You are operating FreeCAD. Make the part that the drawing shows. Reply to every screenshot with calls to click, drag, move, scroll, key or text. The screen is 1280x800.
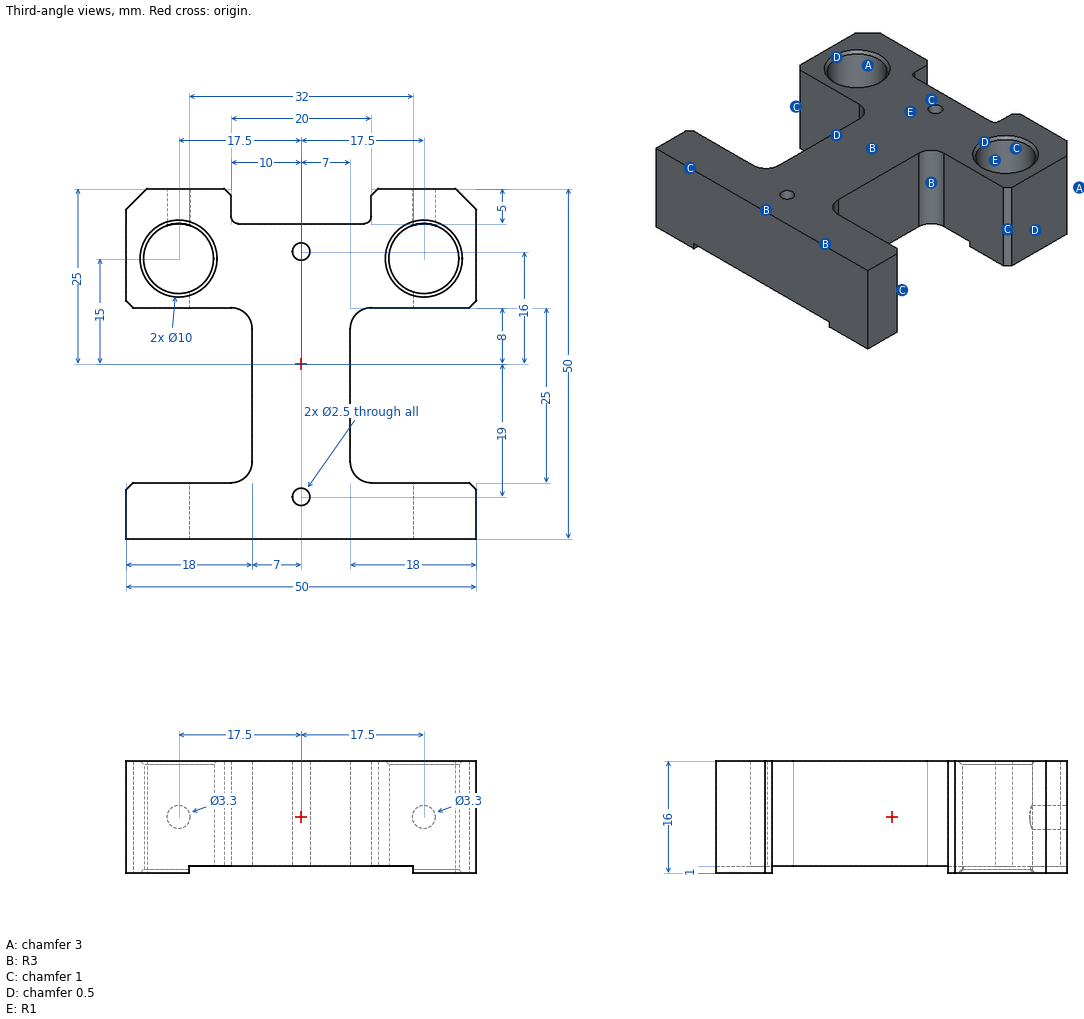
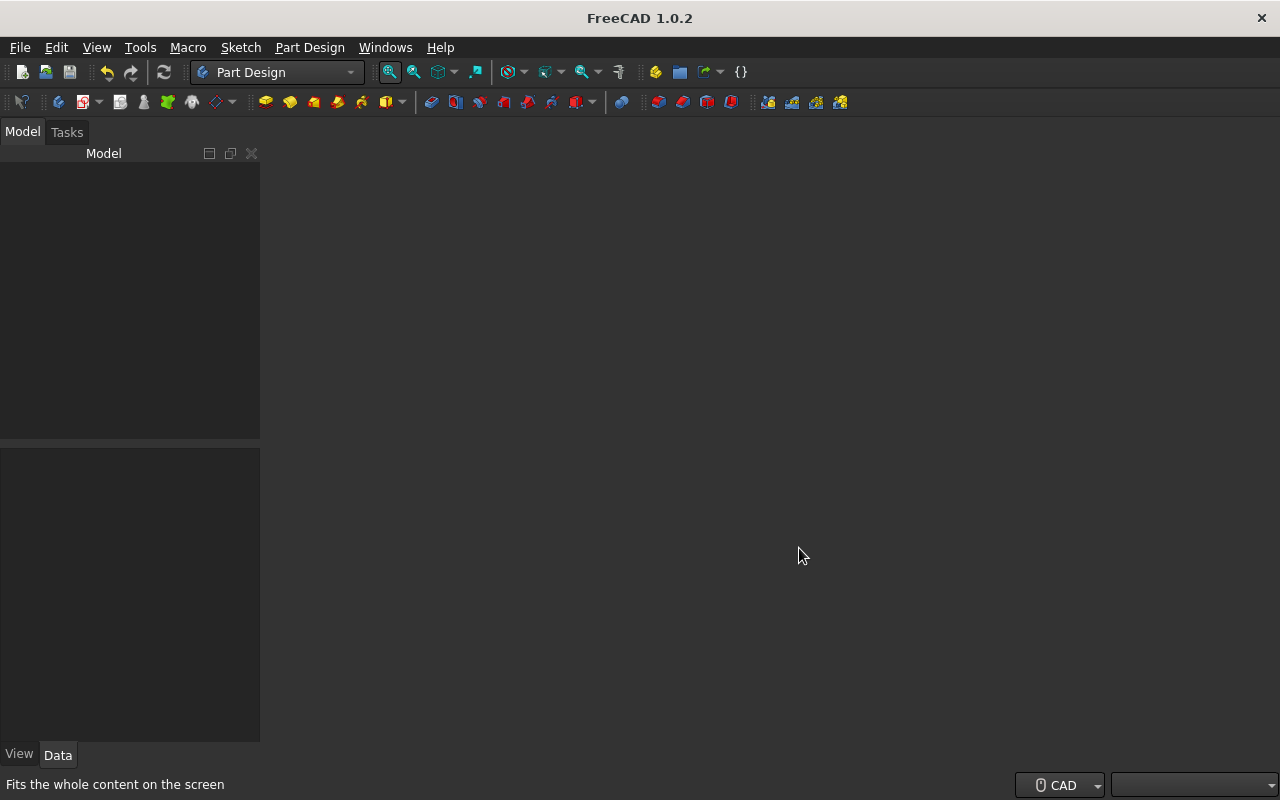
click(22, 72)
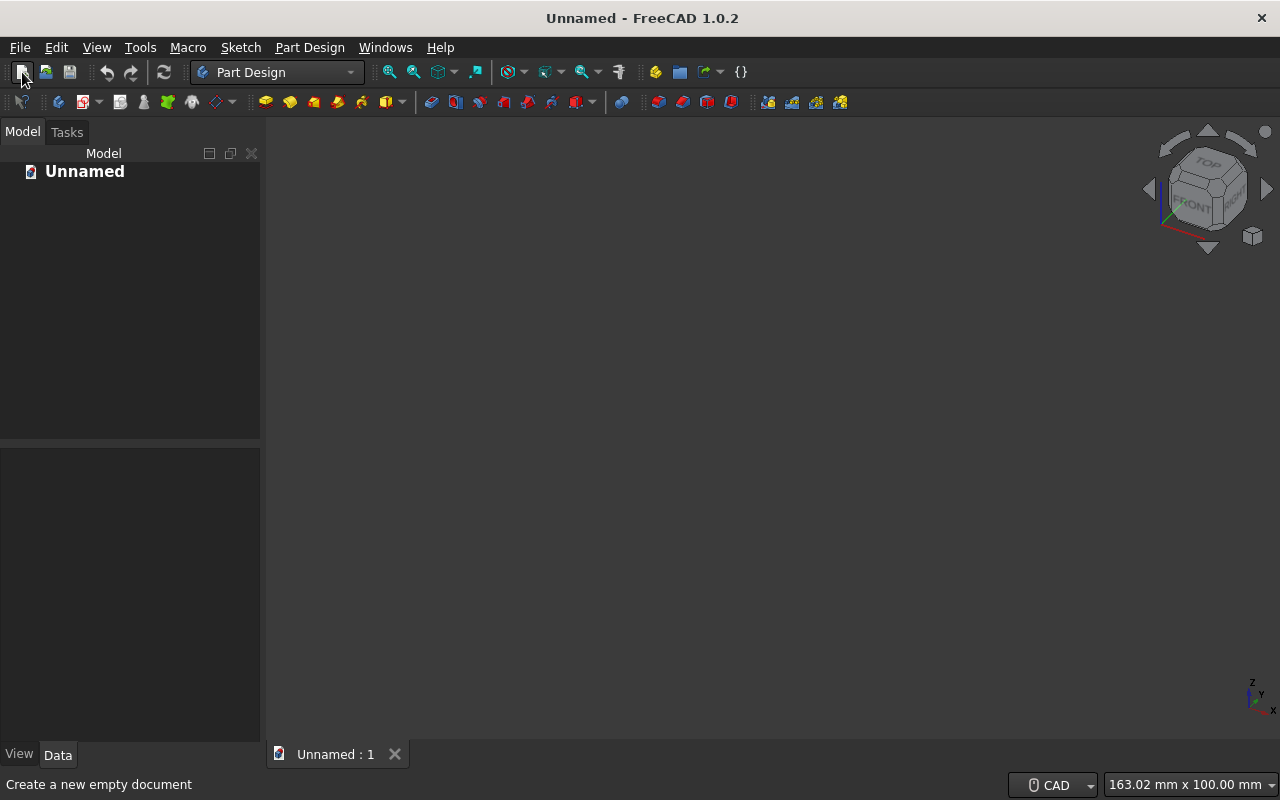
click(84, 102)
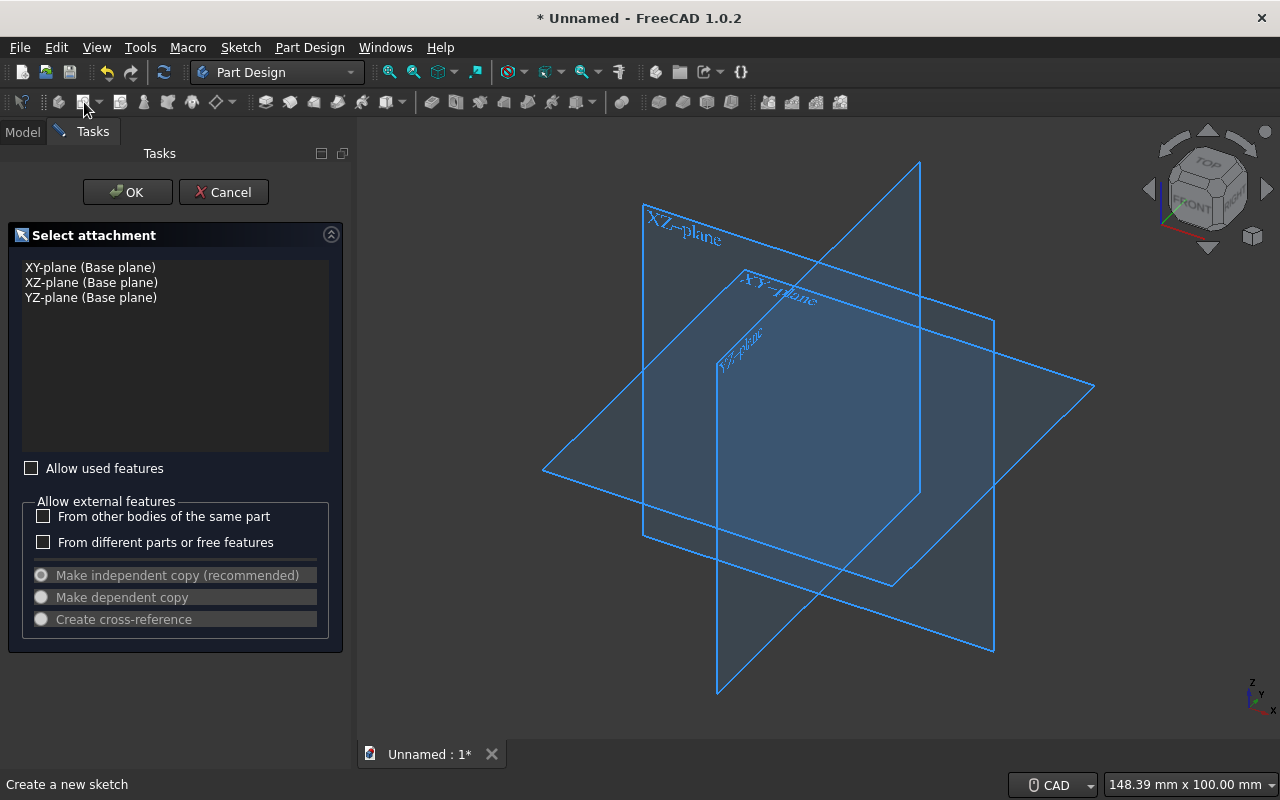
click(82, 268)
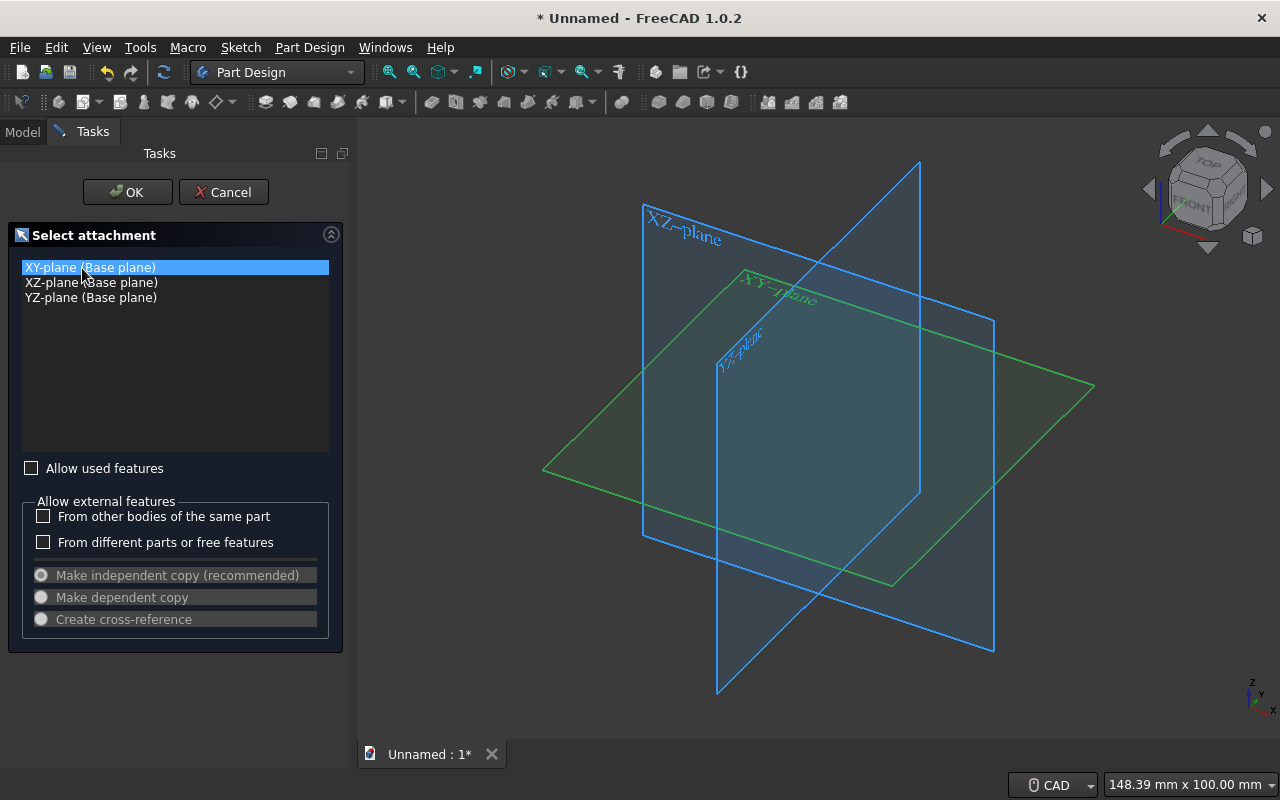
click(128, 192)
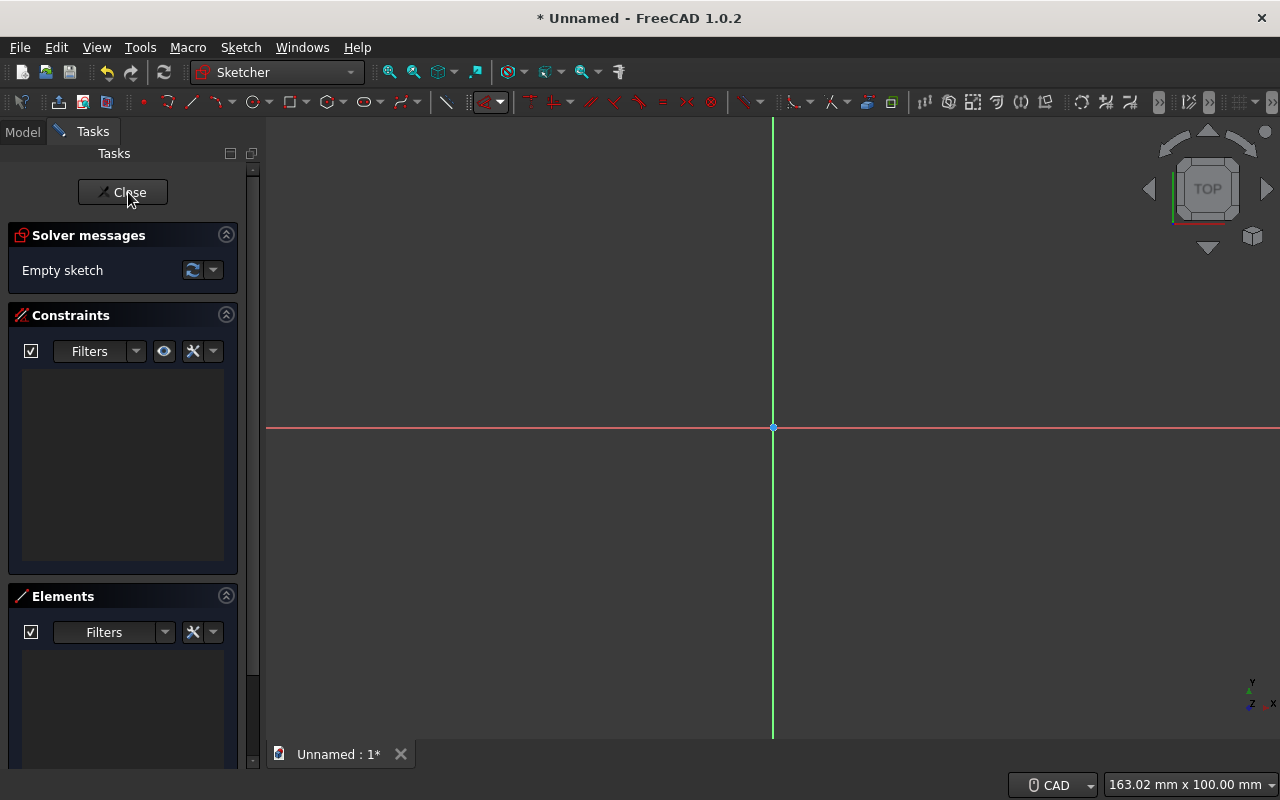
key(g)
key(v)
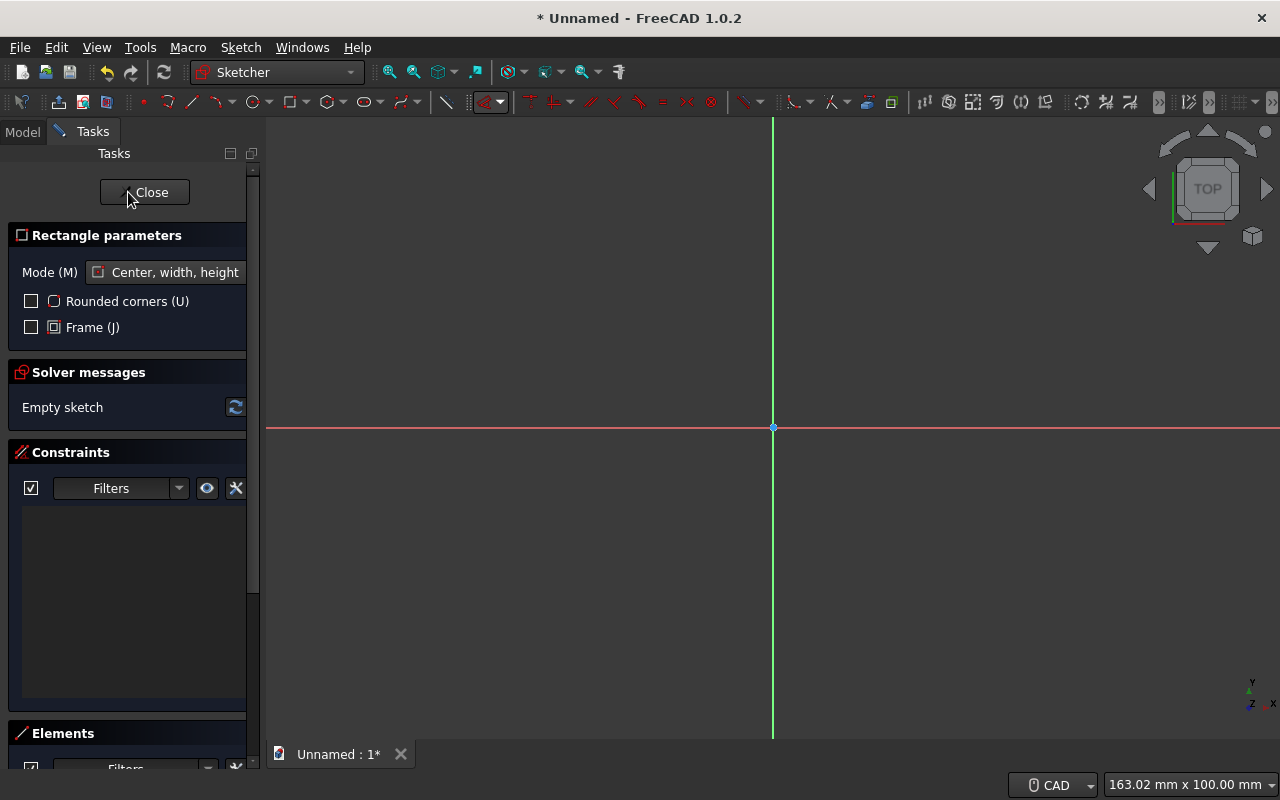
click(773, 428)
move(928, 272)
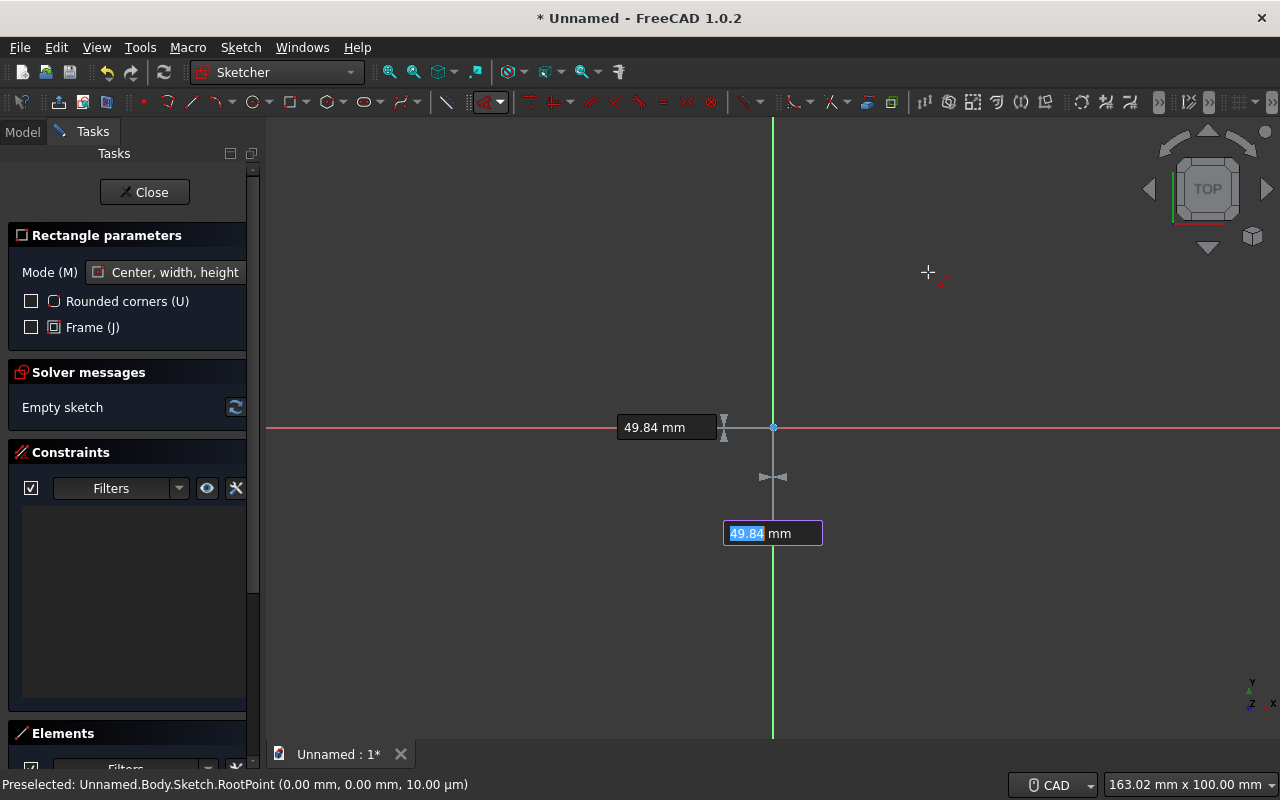
text(50)
key(Tab)
text(50)
key(Return)
key(Escape)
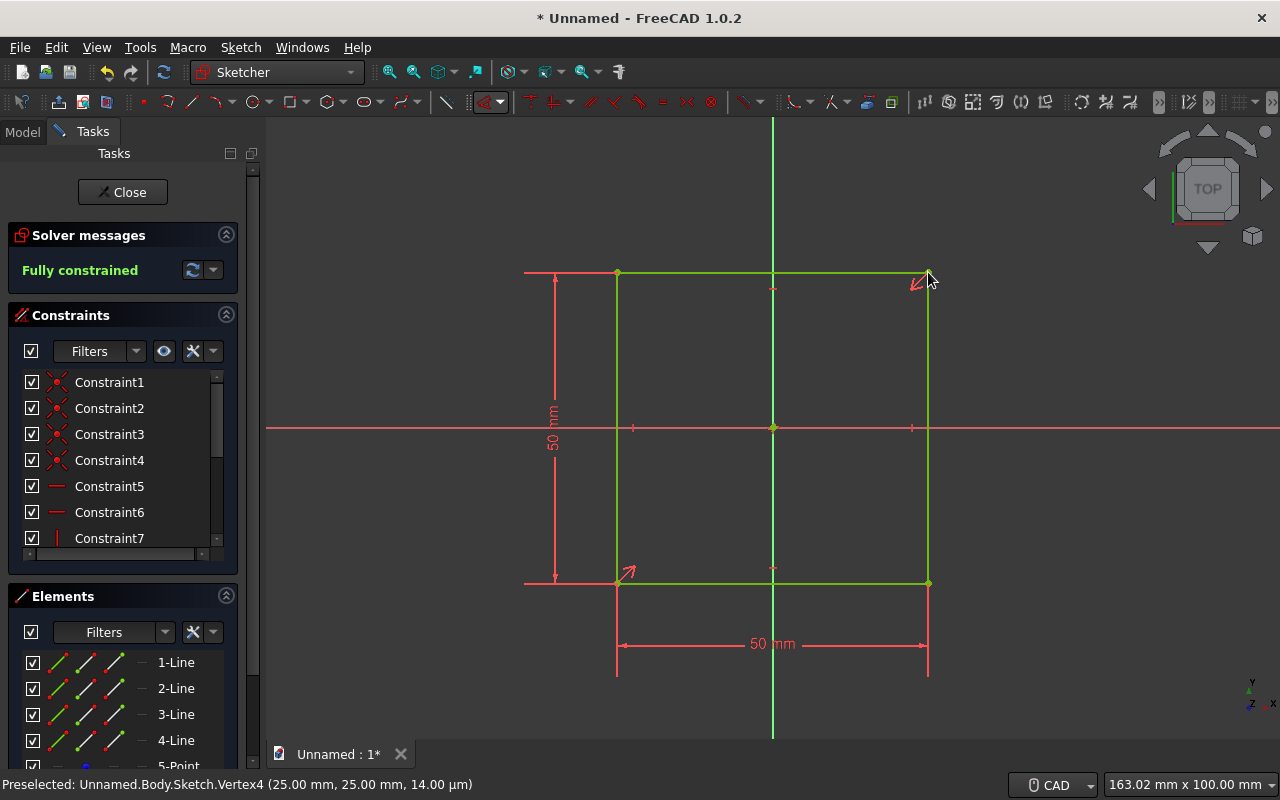
click(123, 192)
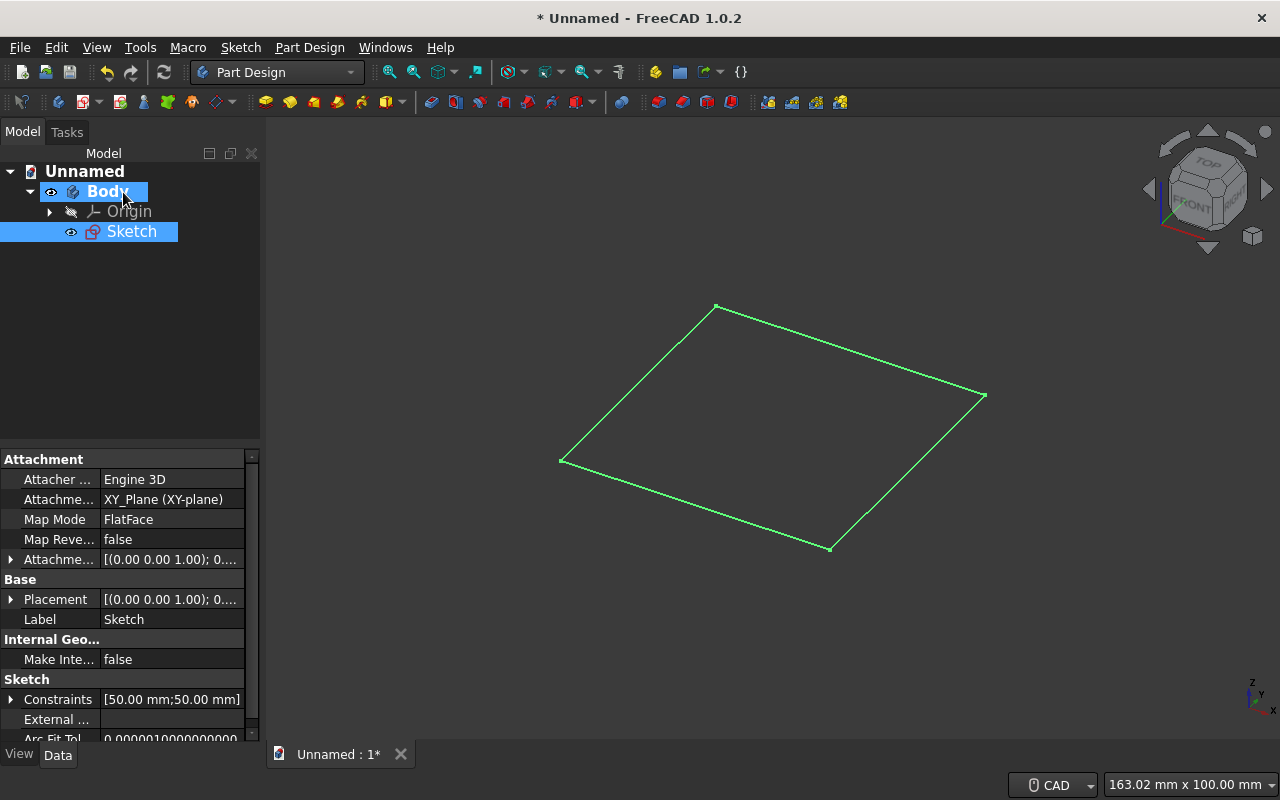
click(266, 102)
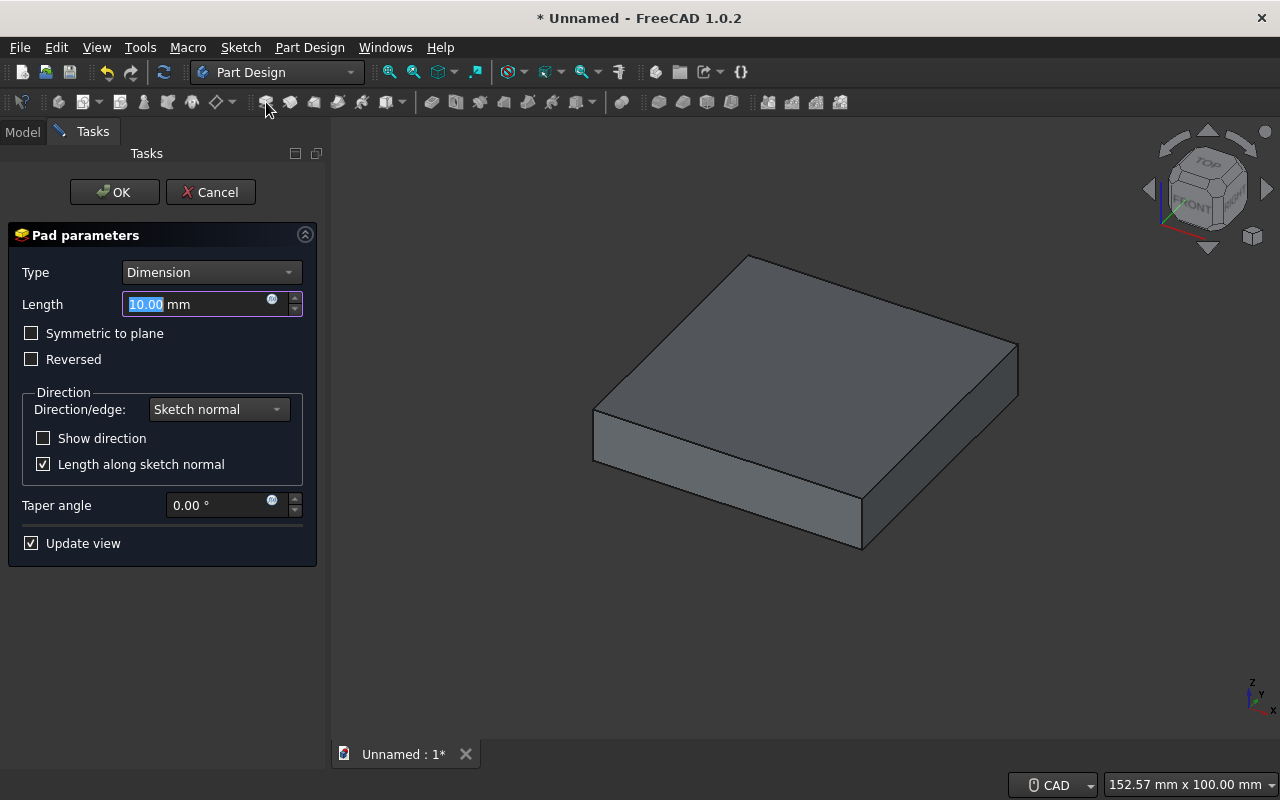
text(16)
key(Tab)